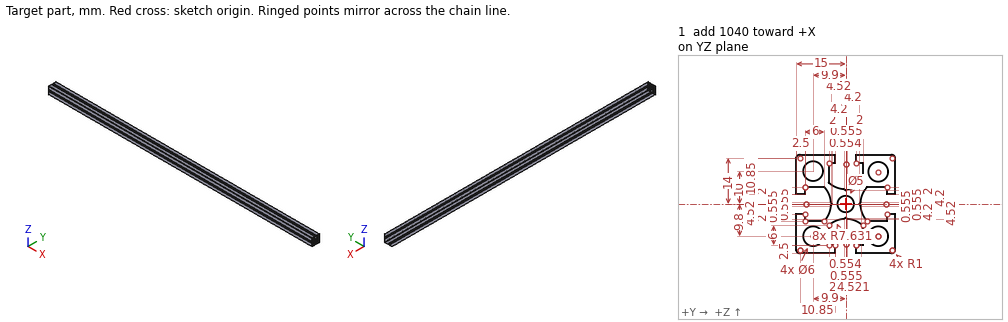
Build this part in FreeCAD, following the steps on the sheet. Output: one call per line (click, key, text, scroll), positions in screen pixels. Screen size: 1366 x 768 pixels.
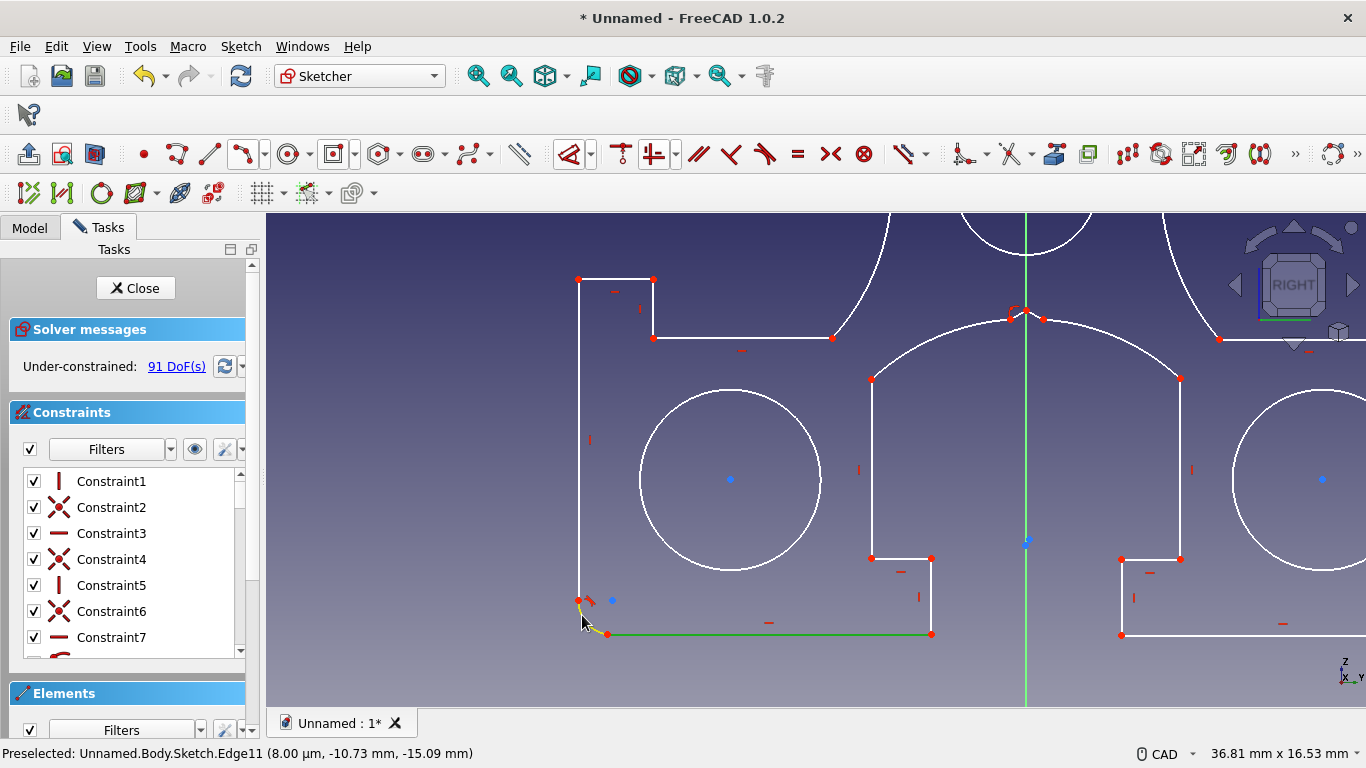
click(582, 615)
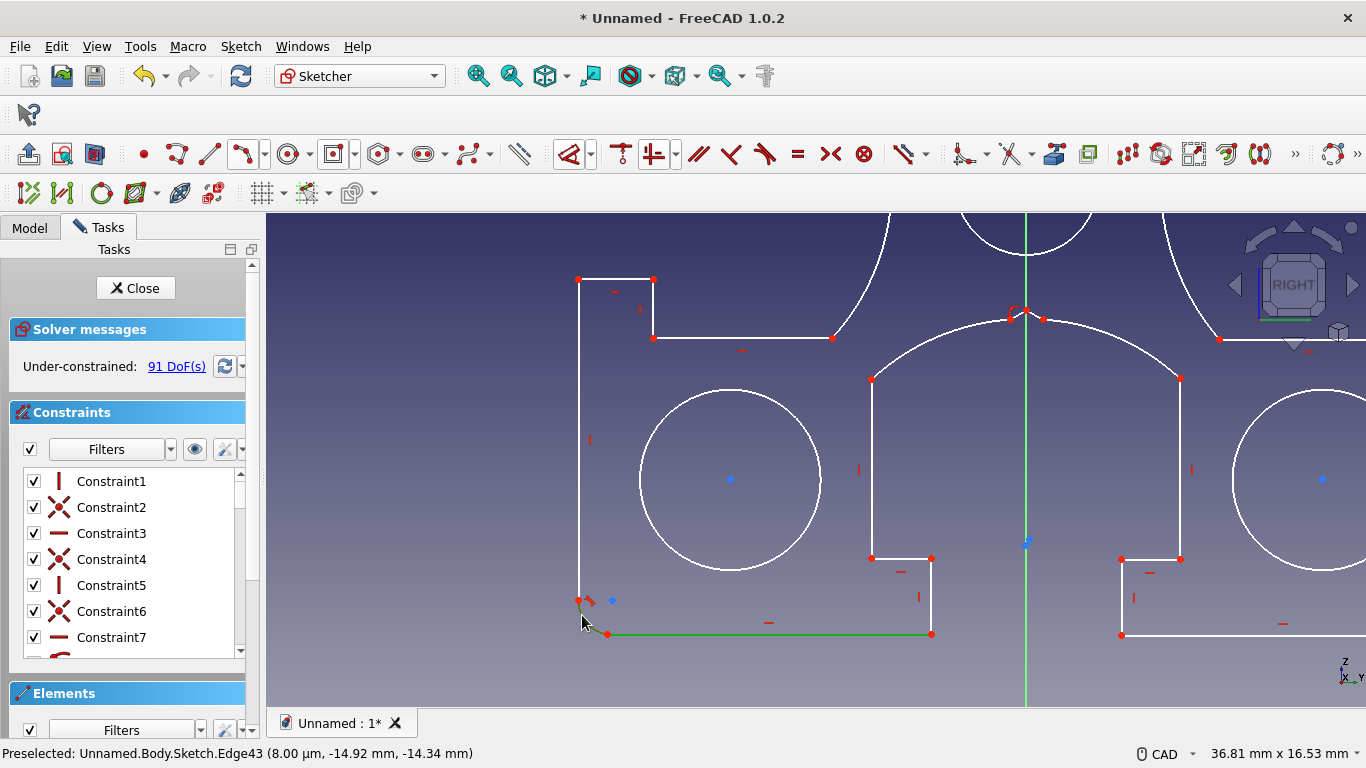
key(t)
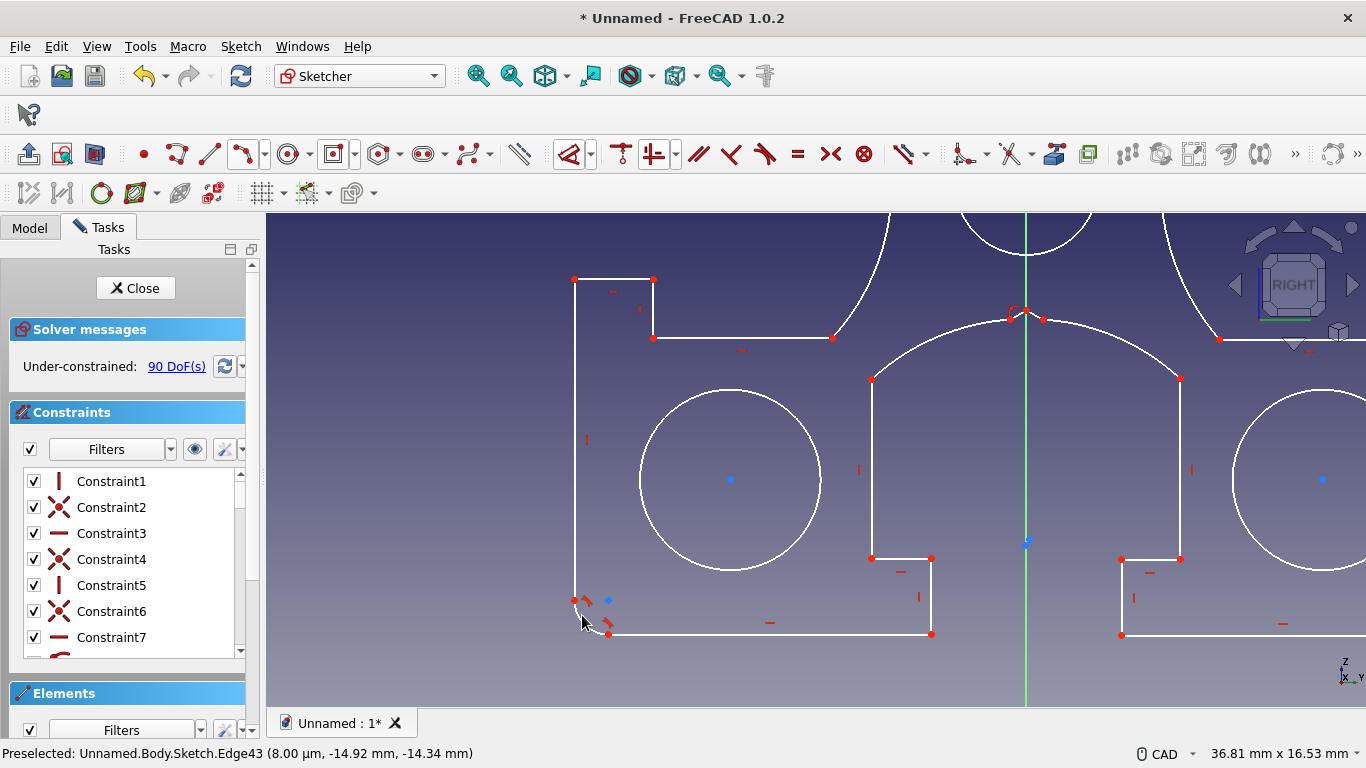
click(1186, 636)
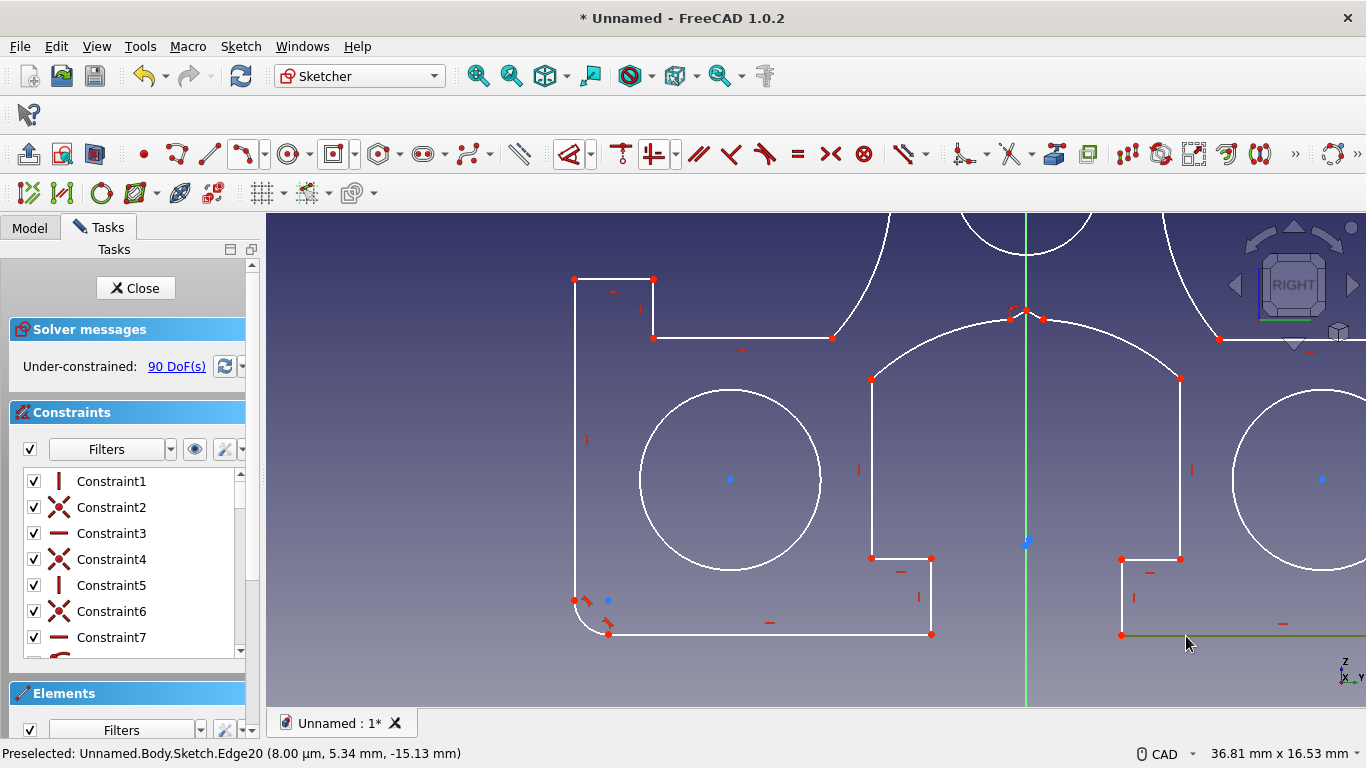
scroll(585, 621, down, 5)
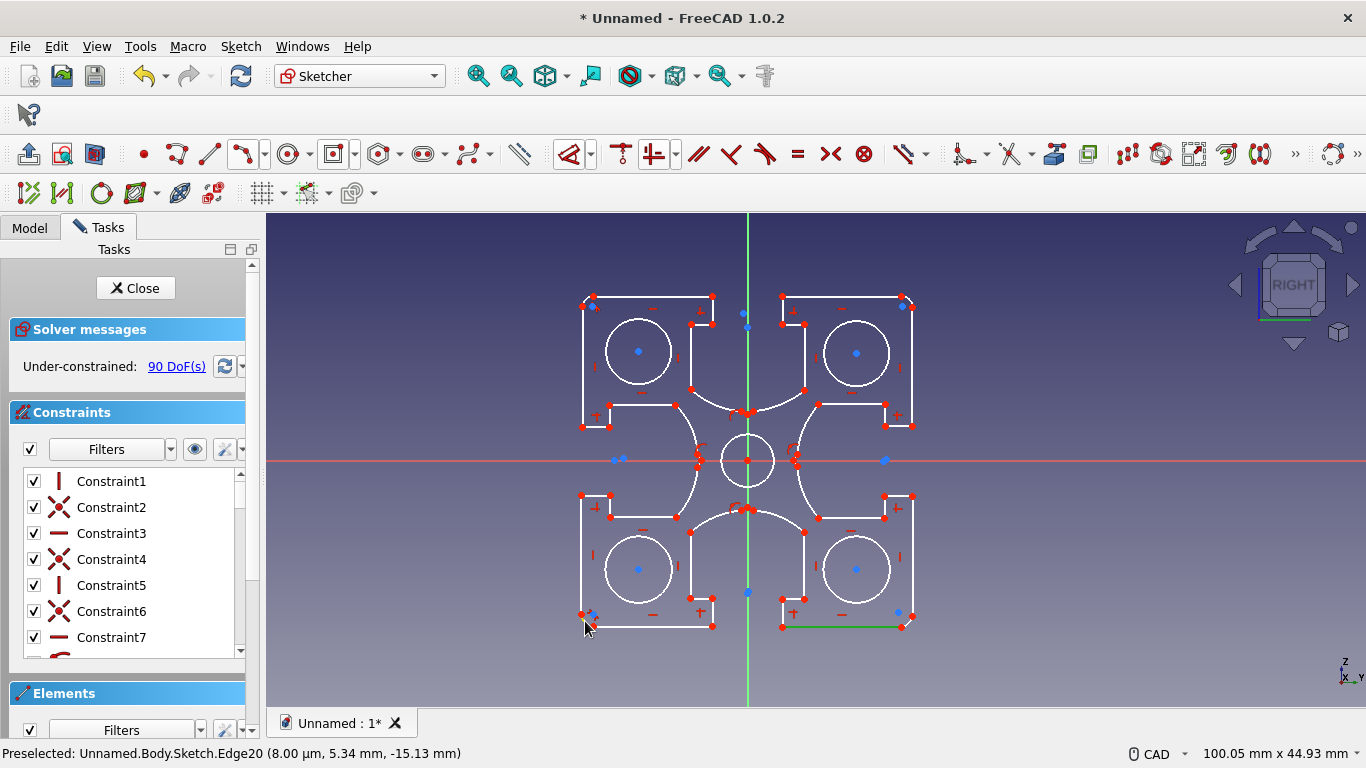
scroll(906, 625, up, 6)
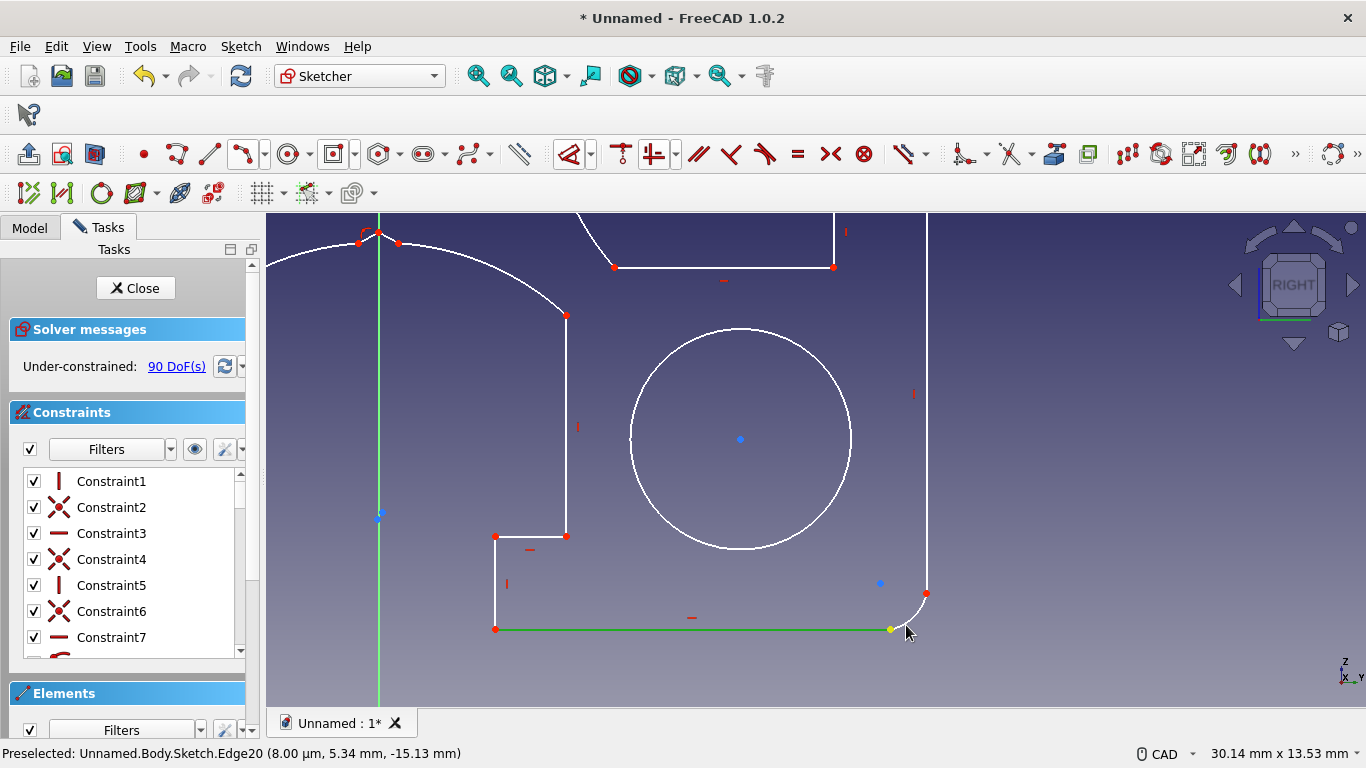
click(905, 624)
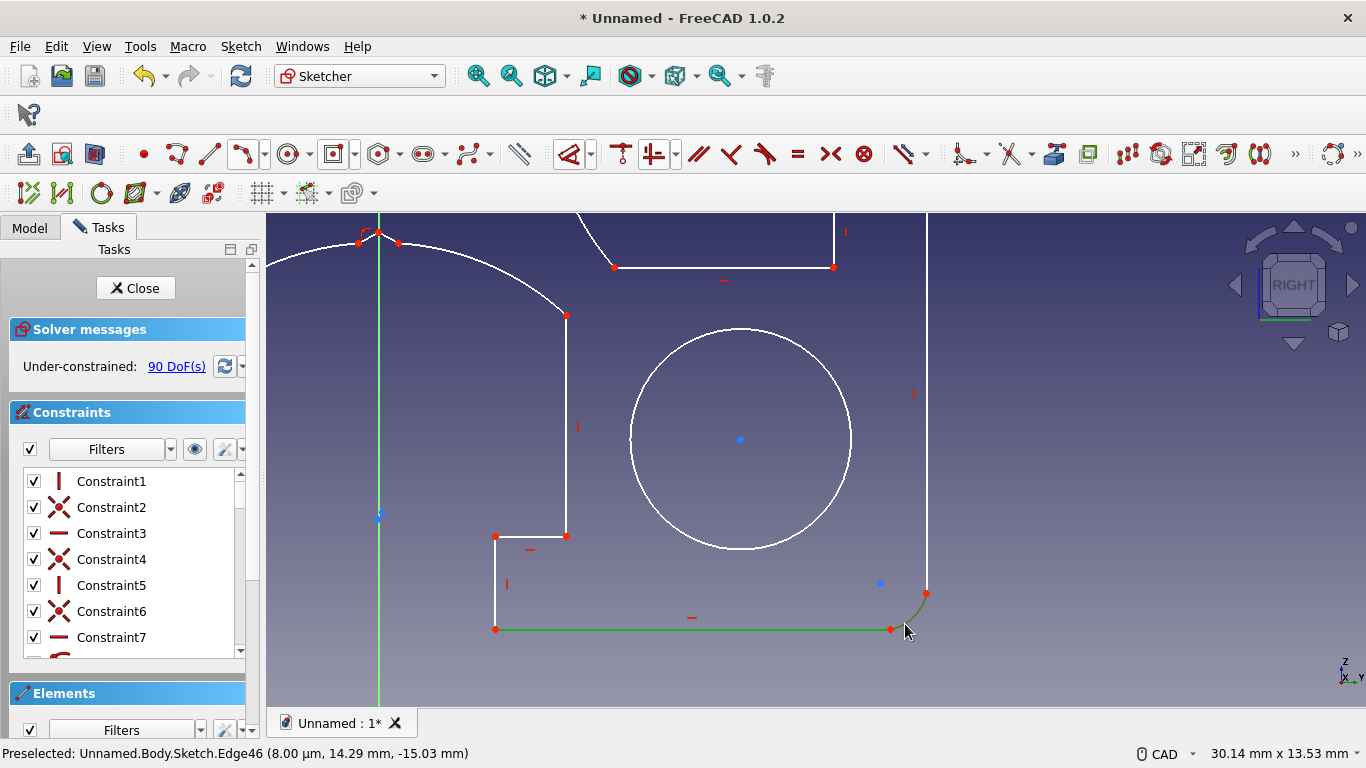
key(t)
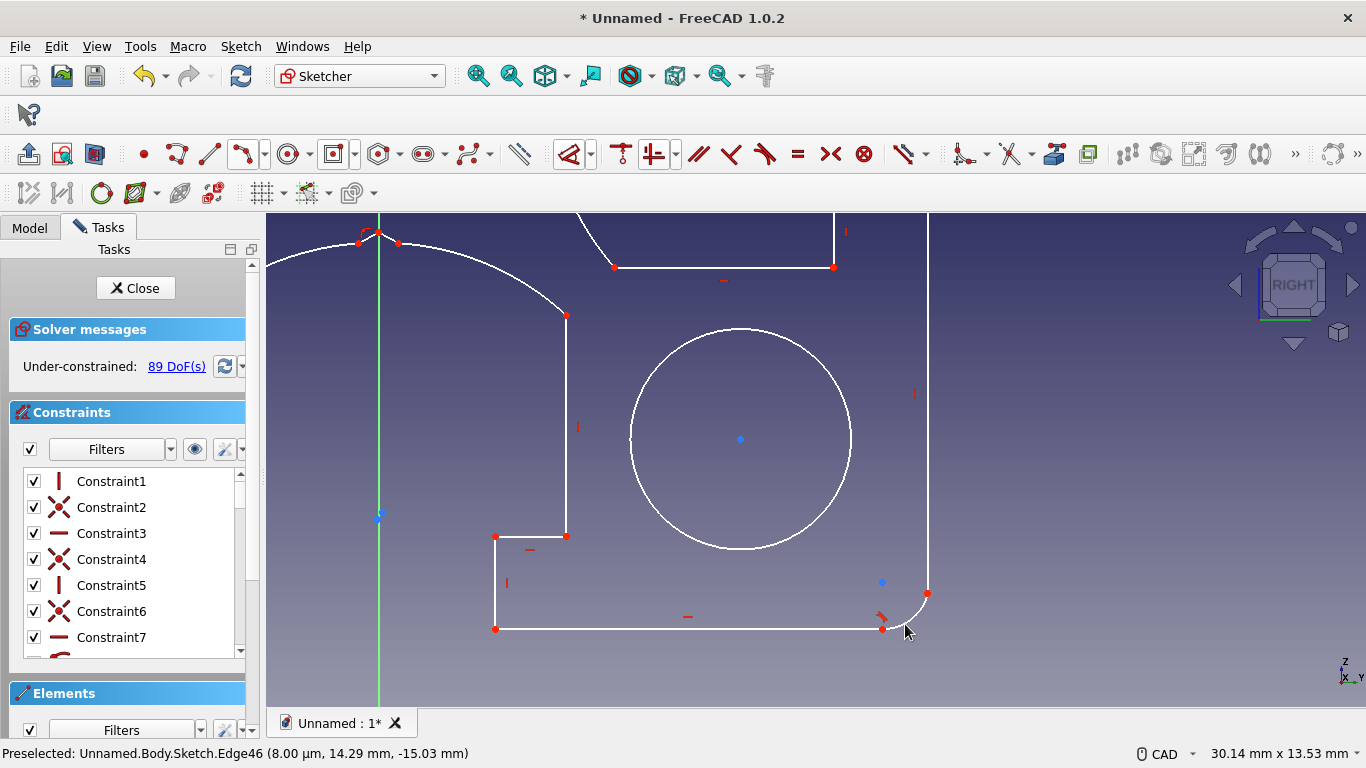
click(928, 474)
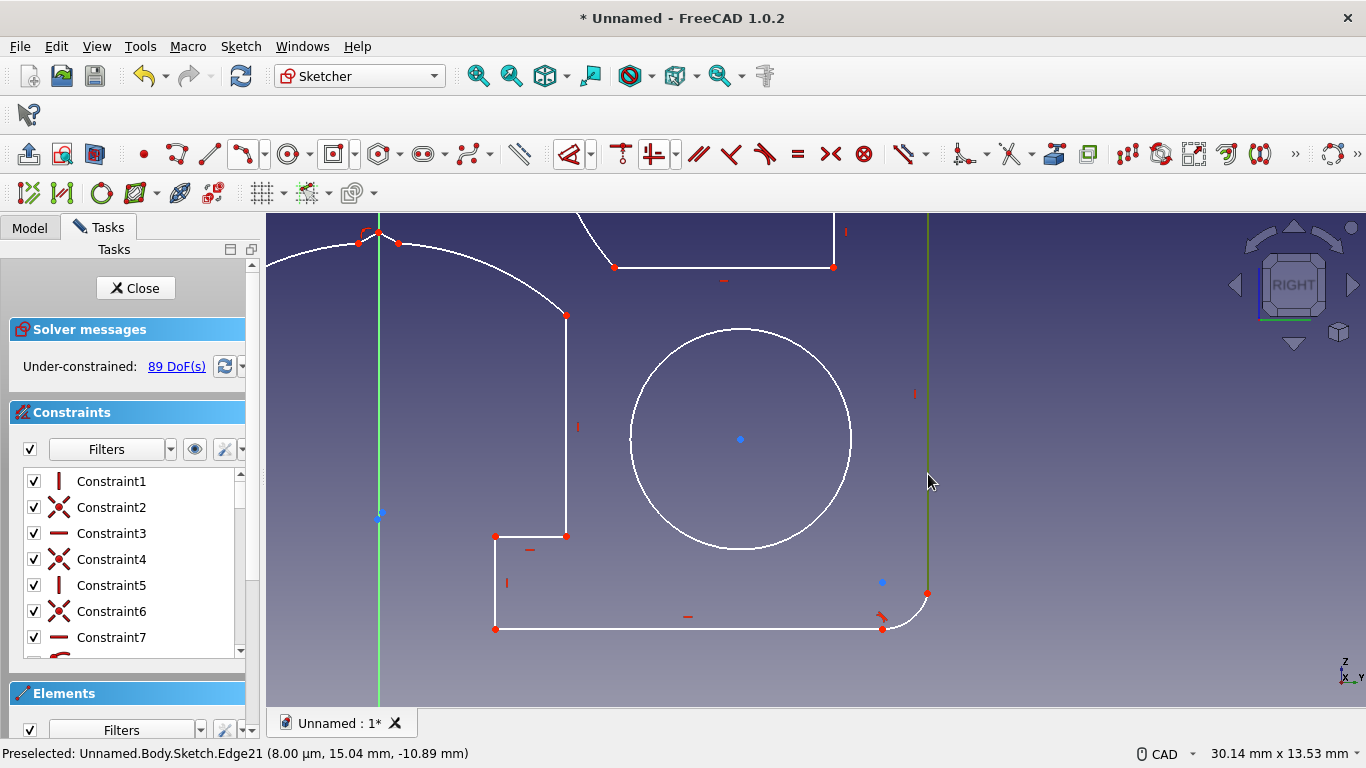
click(901, 625)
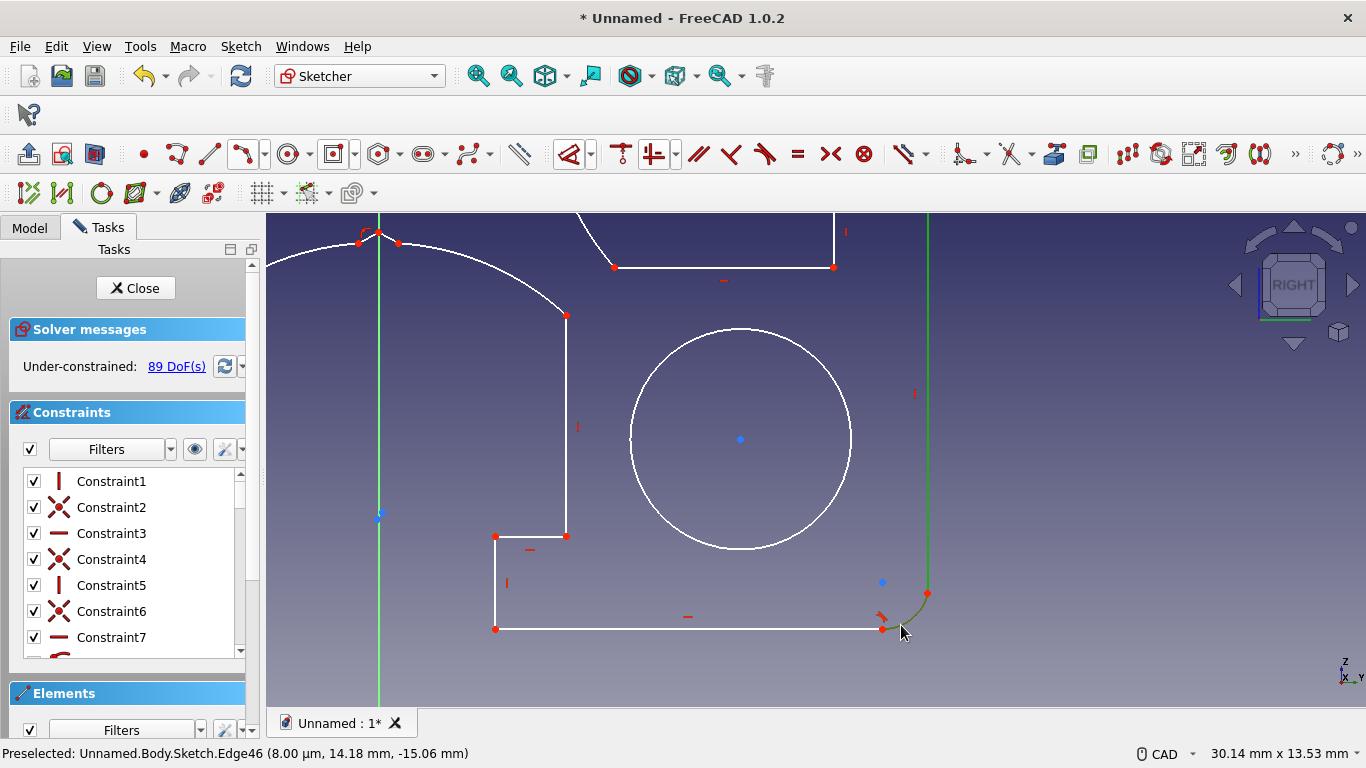
key(t)